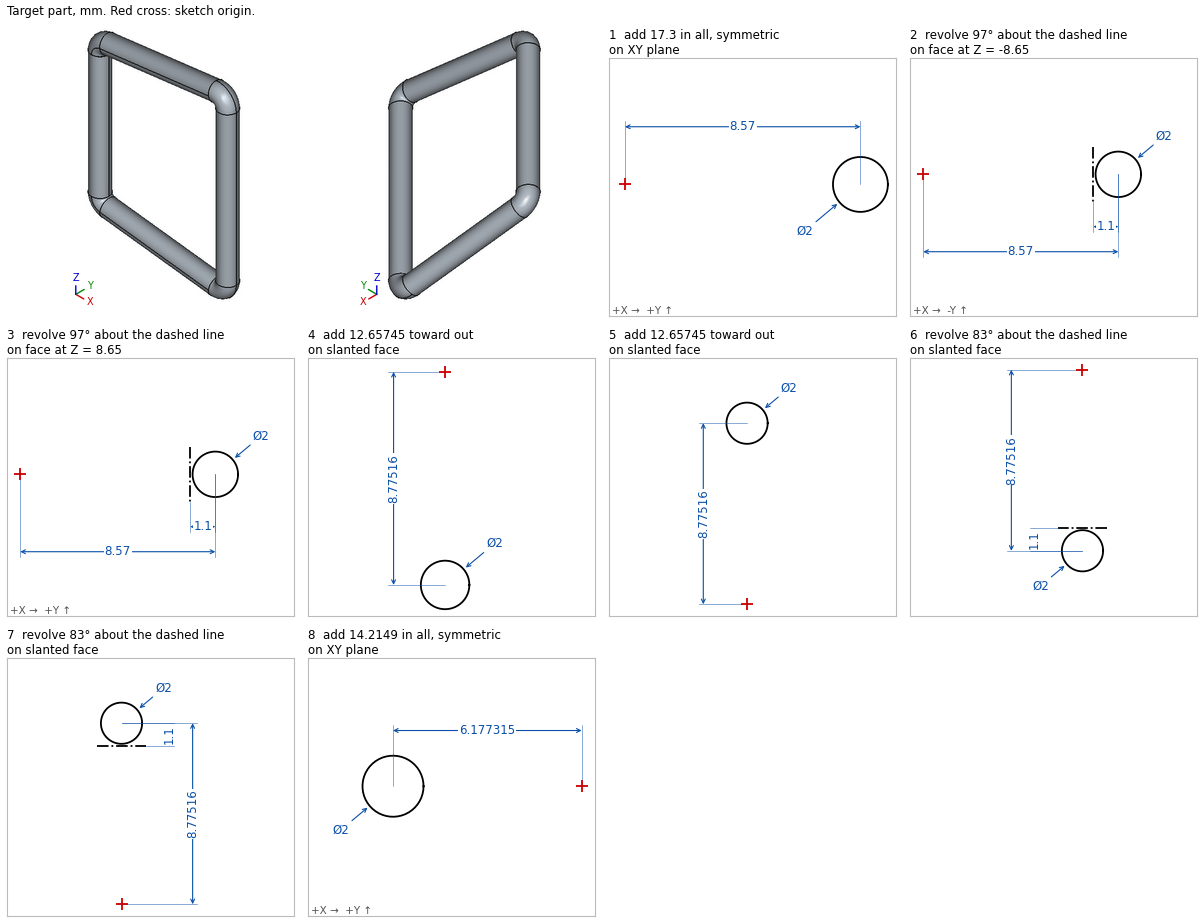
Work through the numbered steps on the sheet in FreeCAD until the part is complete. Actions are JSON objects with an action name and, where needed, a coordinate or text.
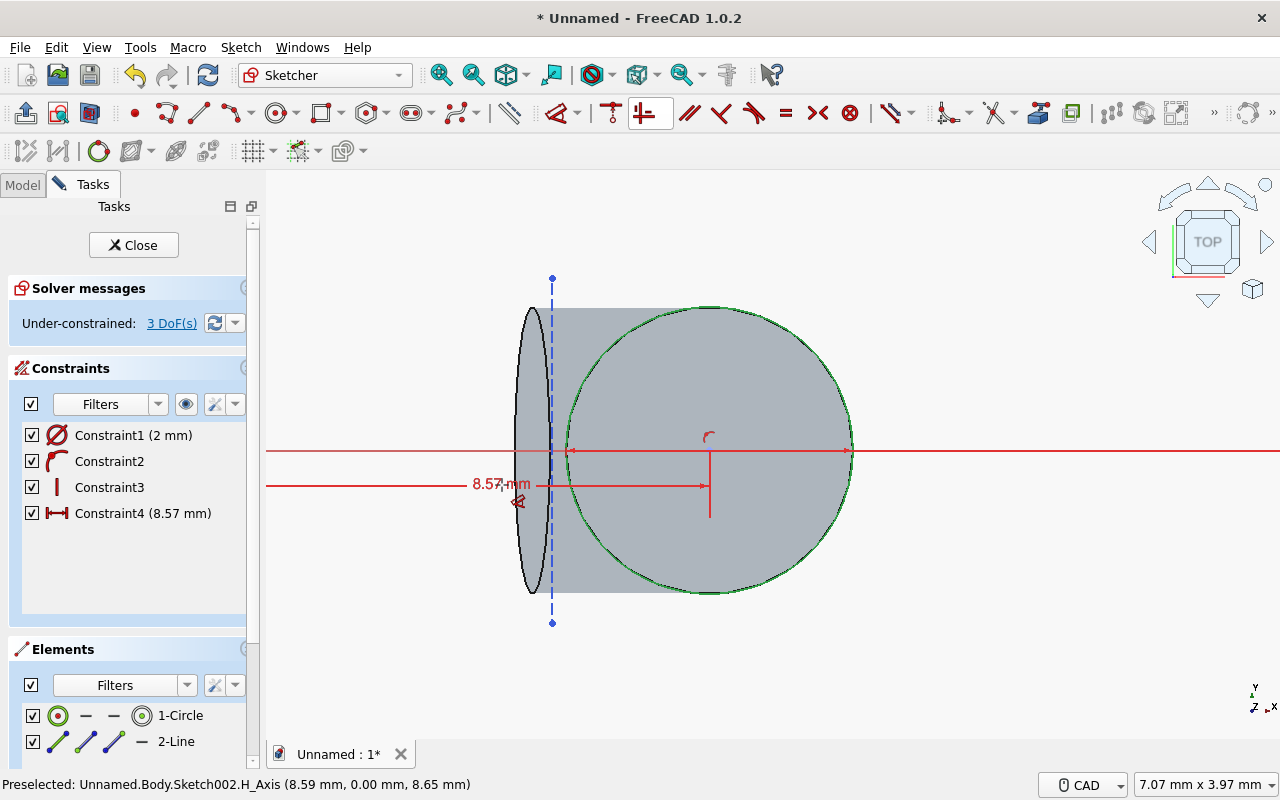
{"action": "left_click", "coordinate": [554, 626]}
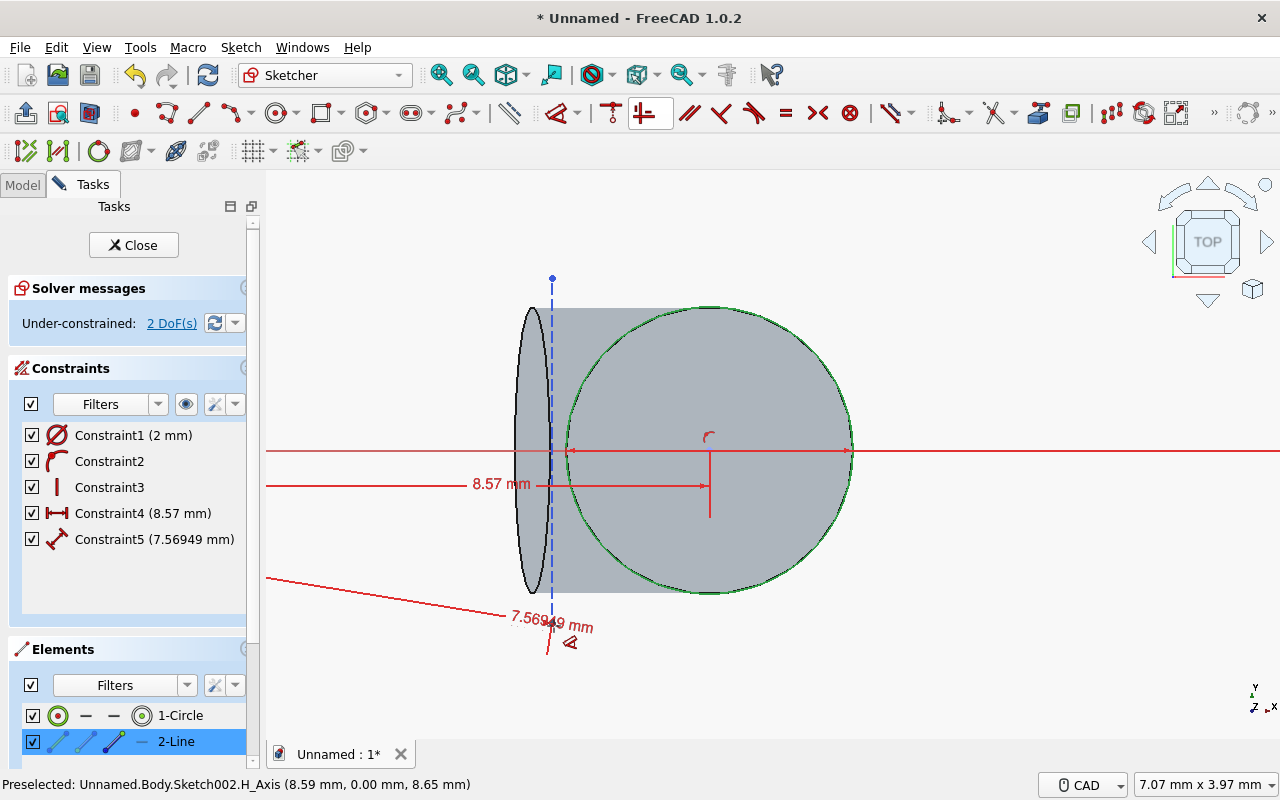
{"action": "left_click", "coordinate": [710, 451]}
{"action": "left_click", "coordinate": [631, 658]}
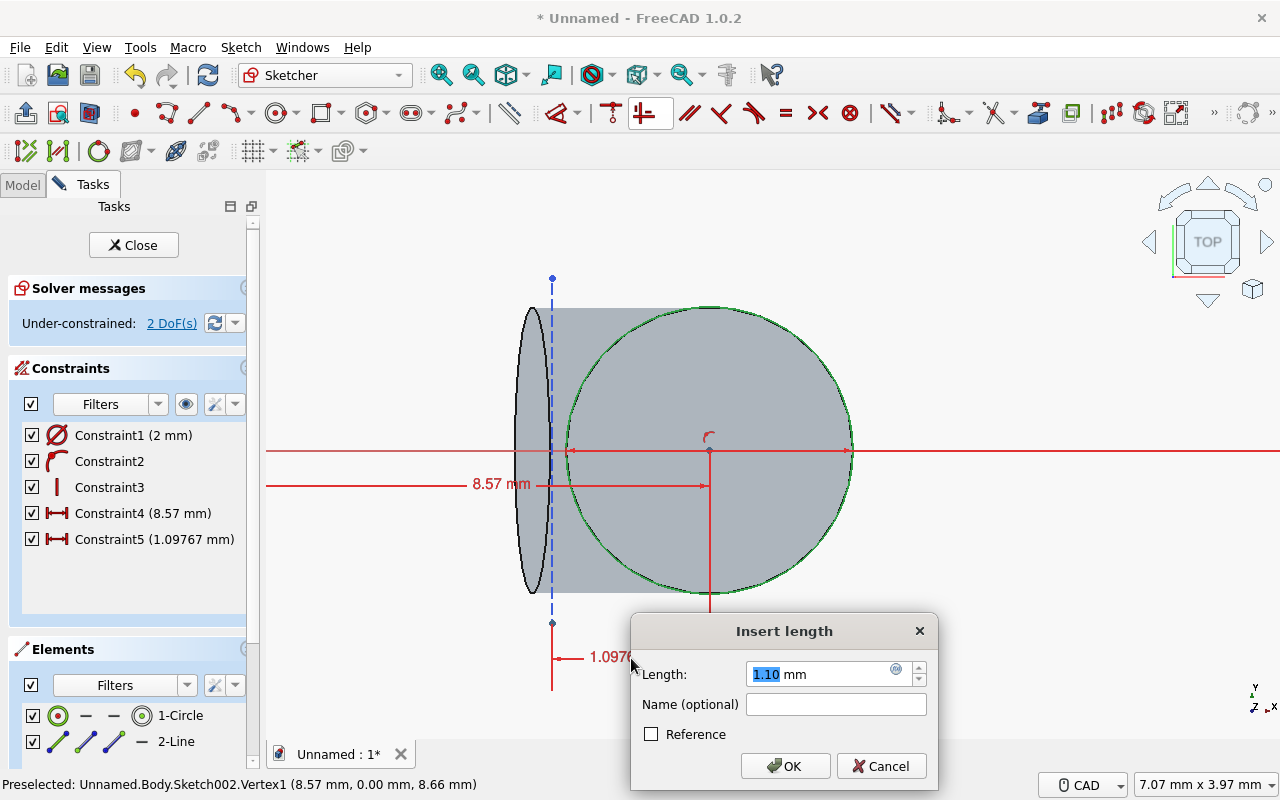
{"action": "type", "text": "1.1"}
{"action": "key", "text": "Return"}
{"action": "key", "text": "Escape"}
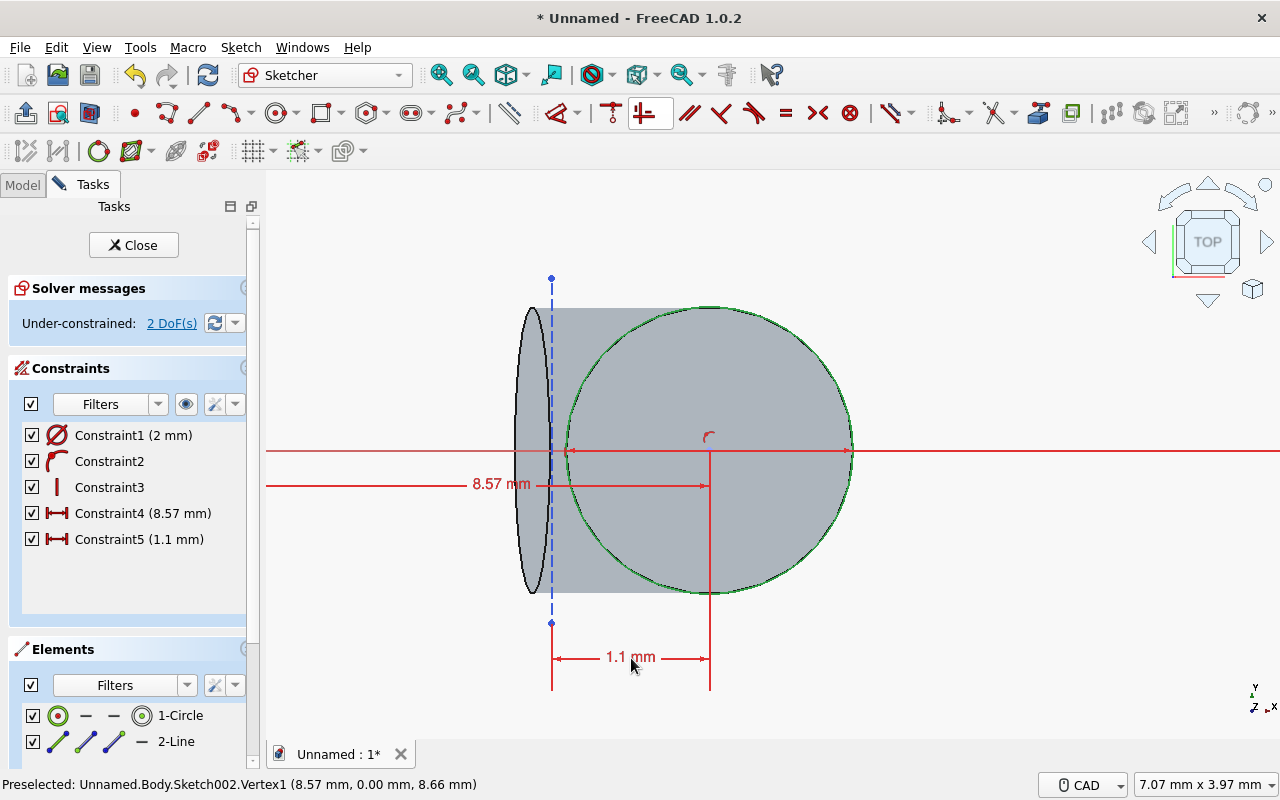
{"action": "left_click", "coordinate": [134, 245]}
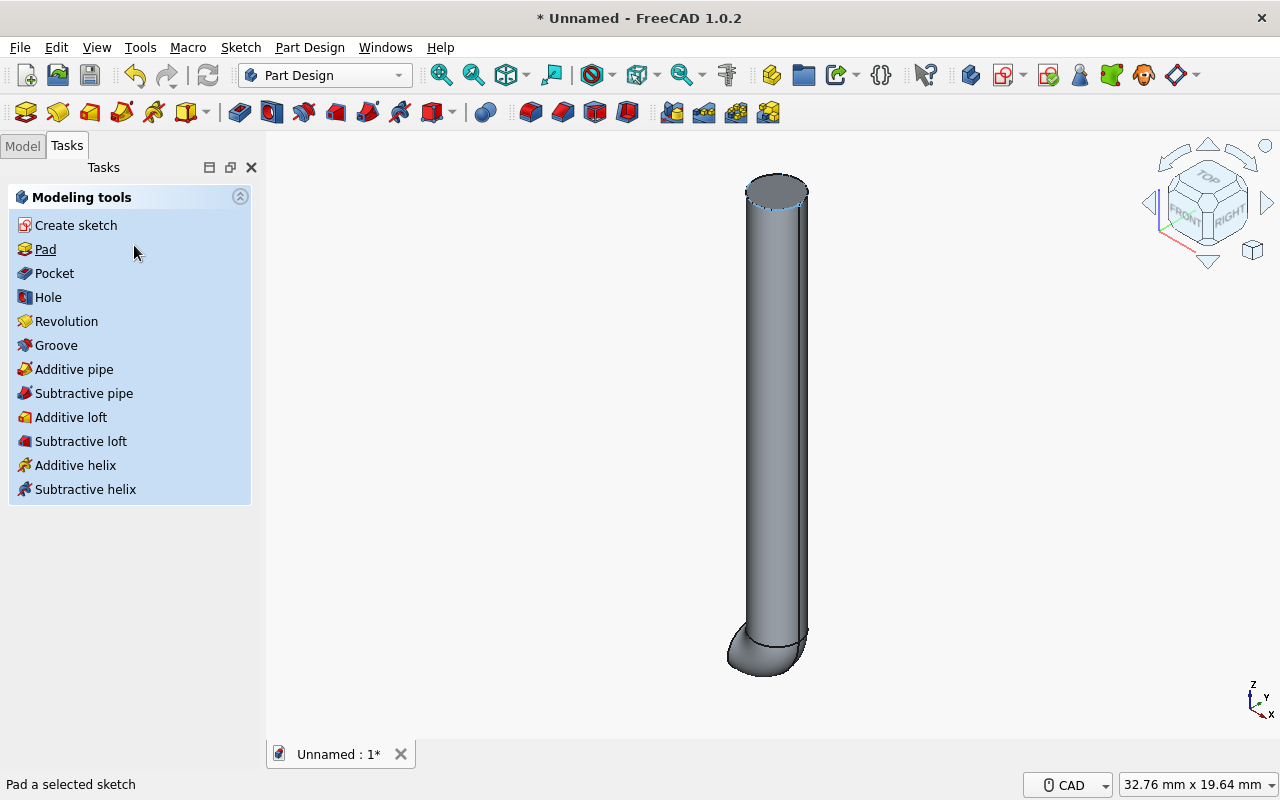
{"action": "left_click", "coordinate": [58, 112]}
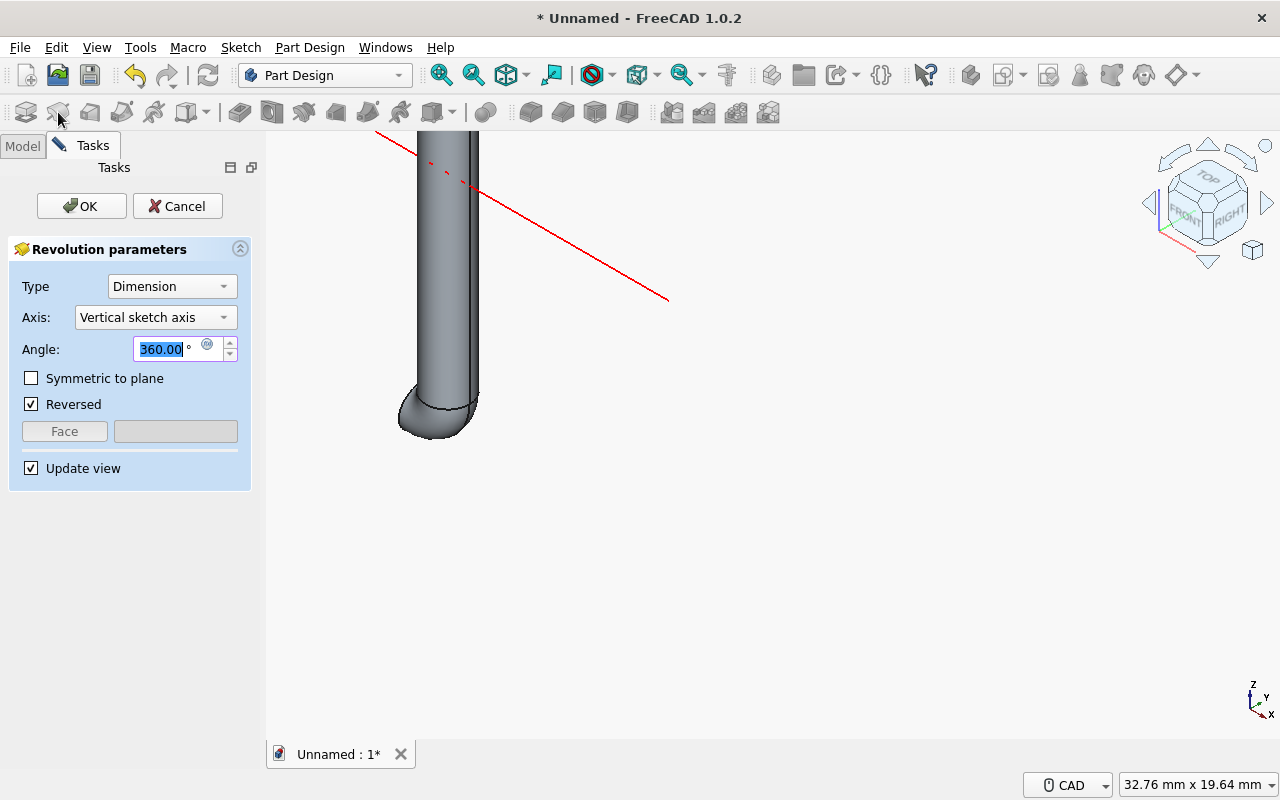
{"action": "left_click", "coordinate": [156, 318]}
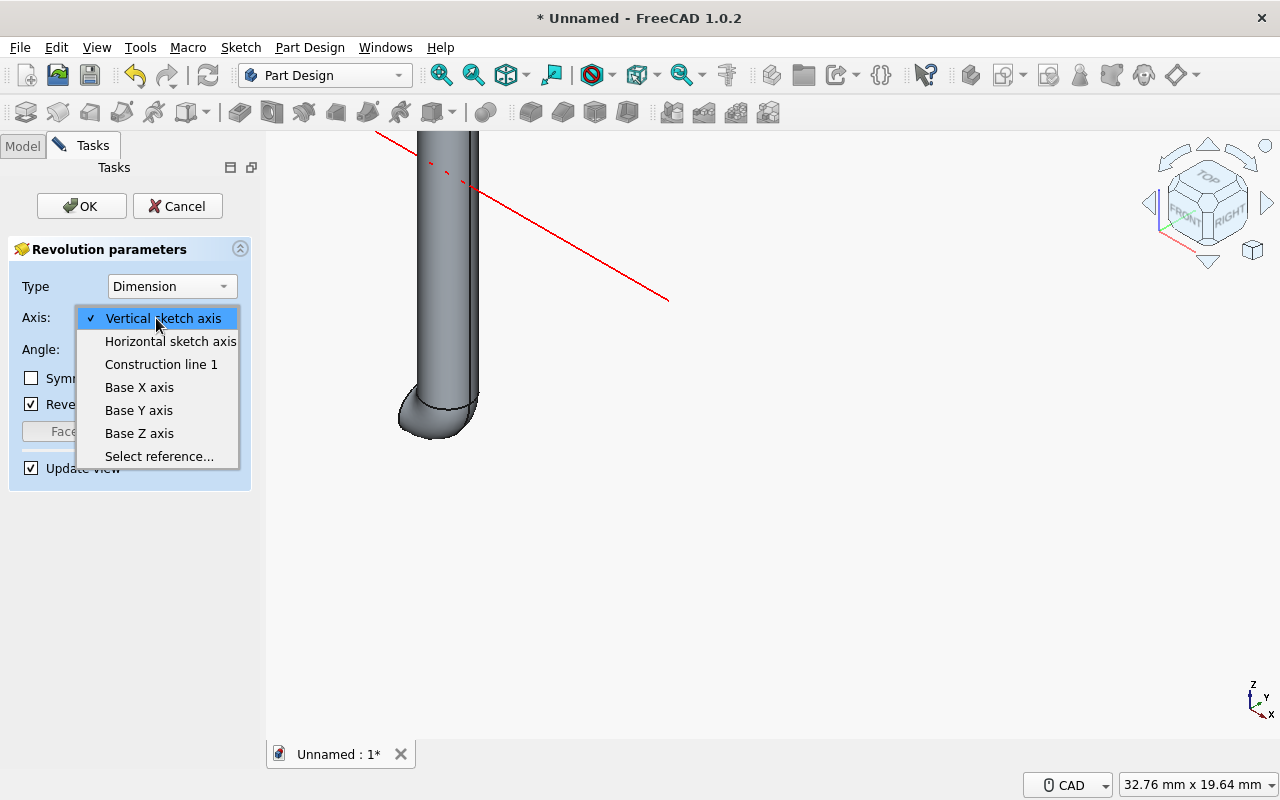
{"action": "left_click", "coordinate": [156, 364]}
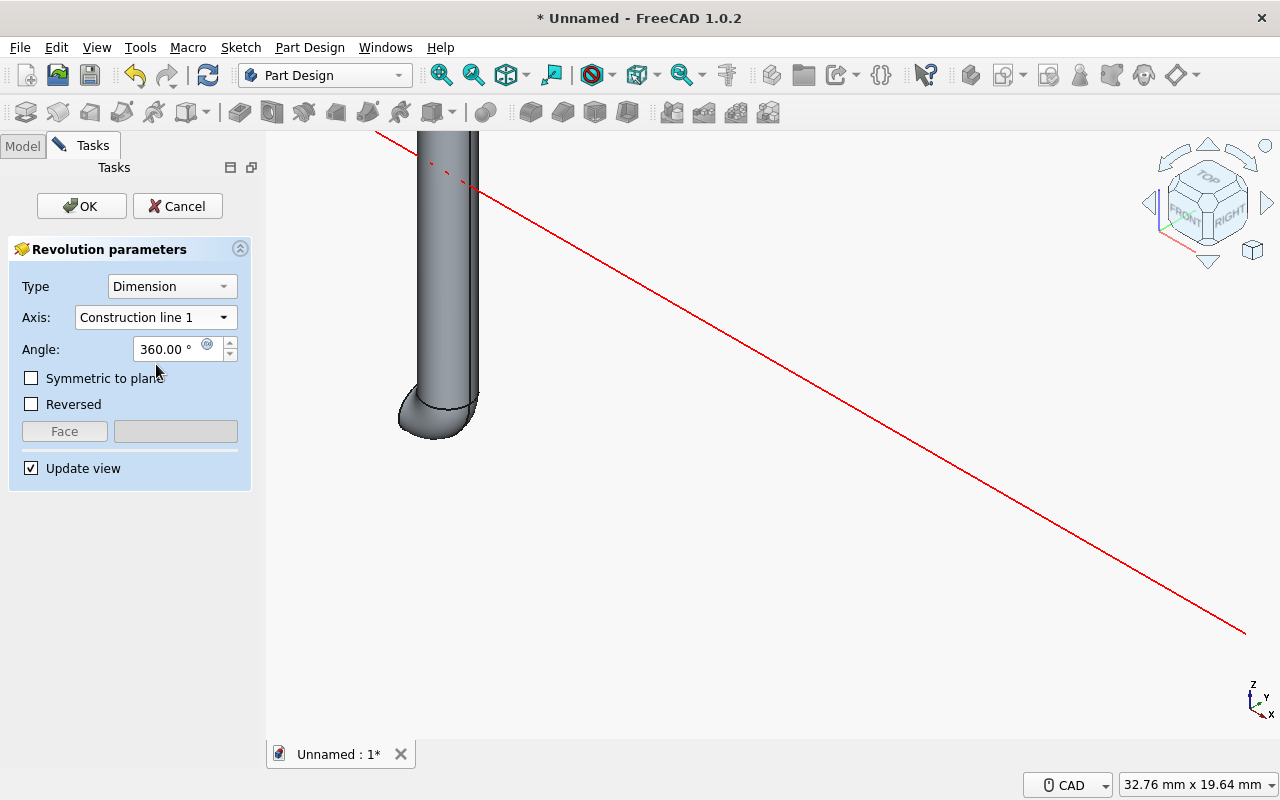
{"action": "triple_click", "coordinate": [178, 349]}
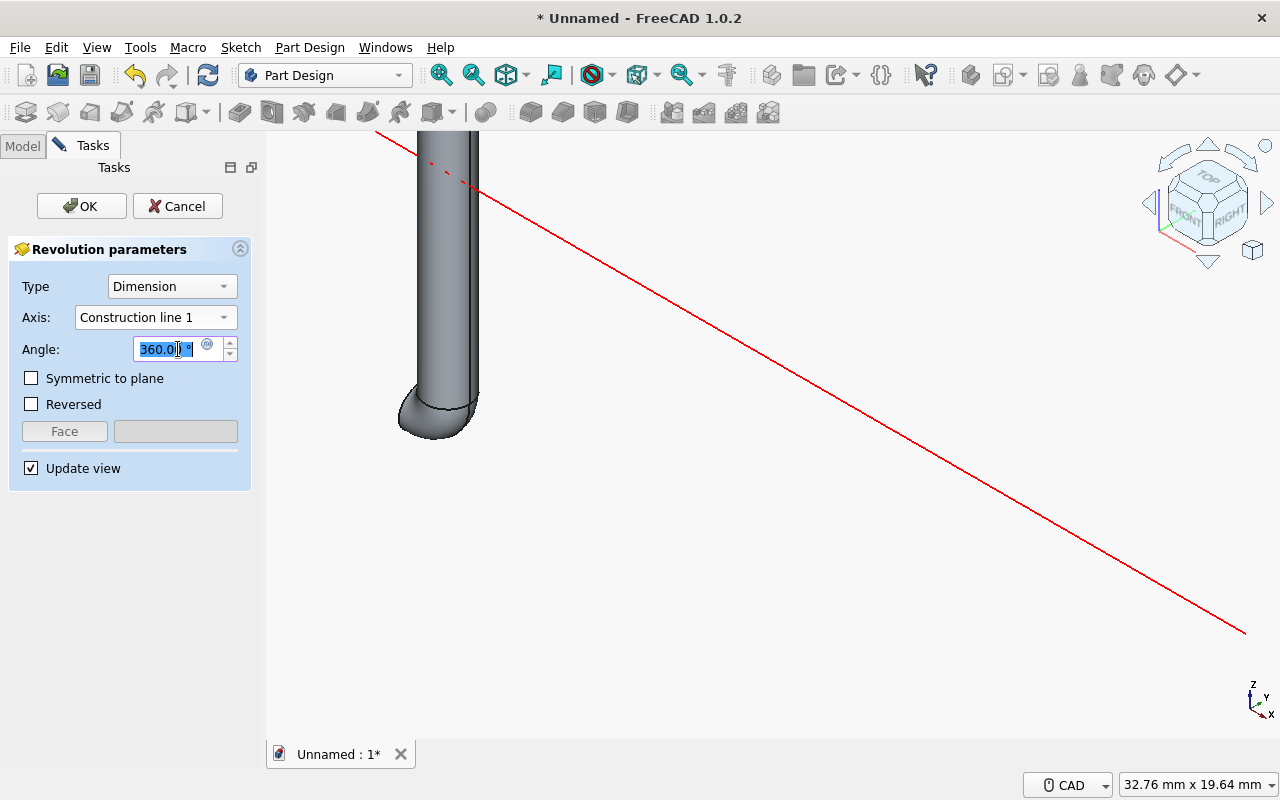
{"action": "type", "text": "97"}
{"action": "key", "text": "Tab"}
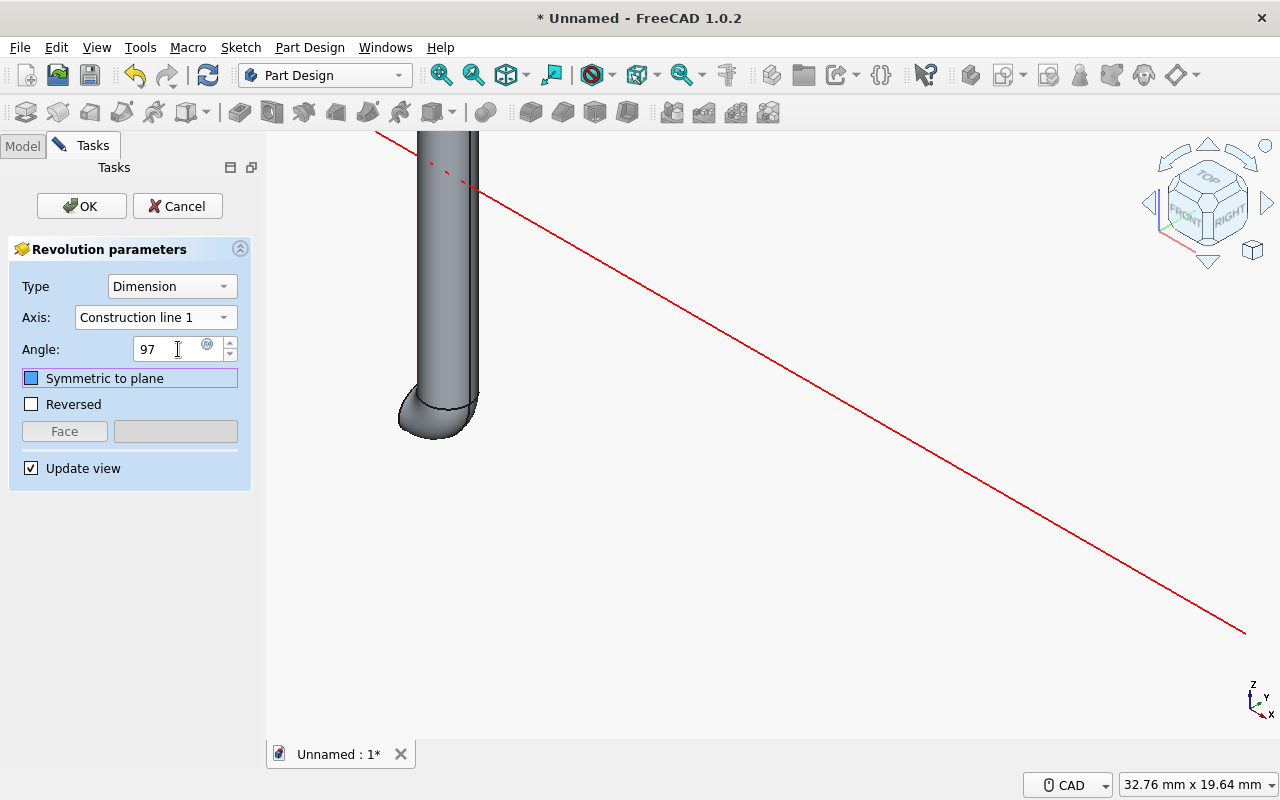
{"action": "left_click", "coordinate": [82, 206]}